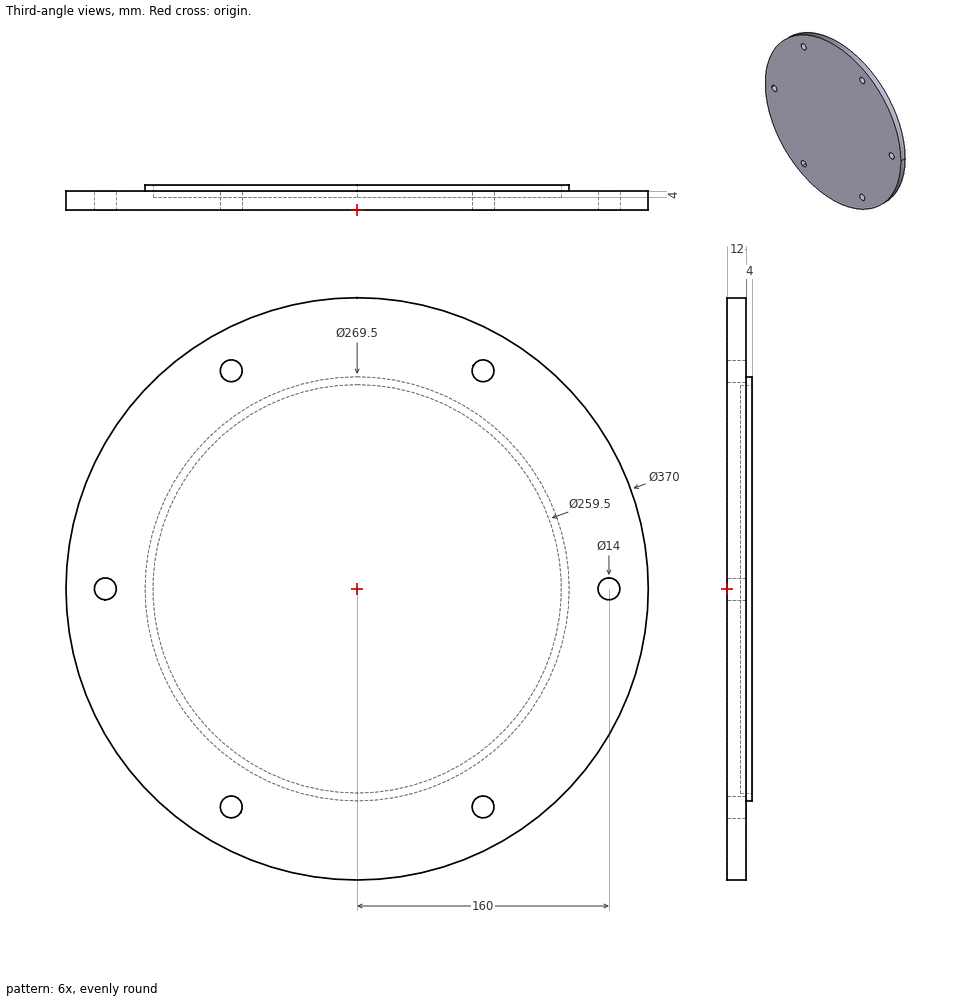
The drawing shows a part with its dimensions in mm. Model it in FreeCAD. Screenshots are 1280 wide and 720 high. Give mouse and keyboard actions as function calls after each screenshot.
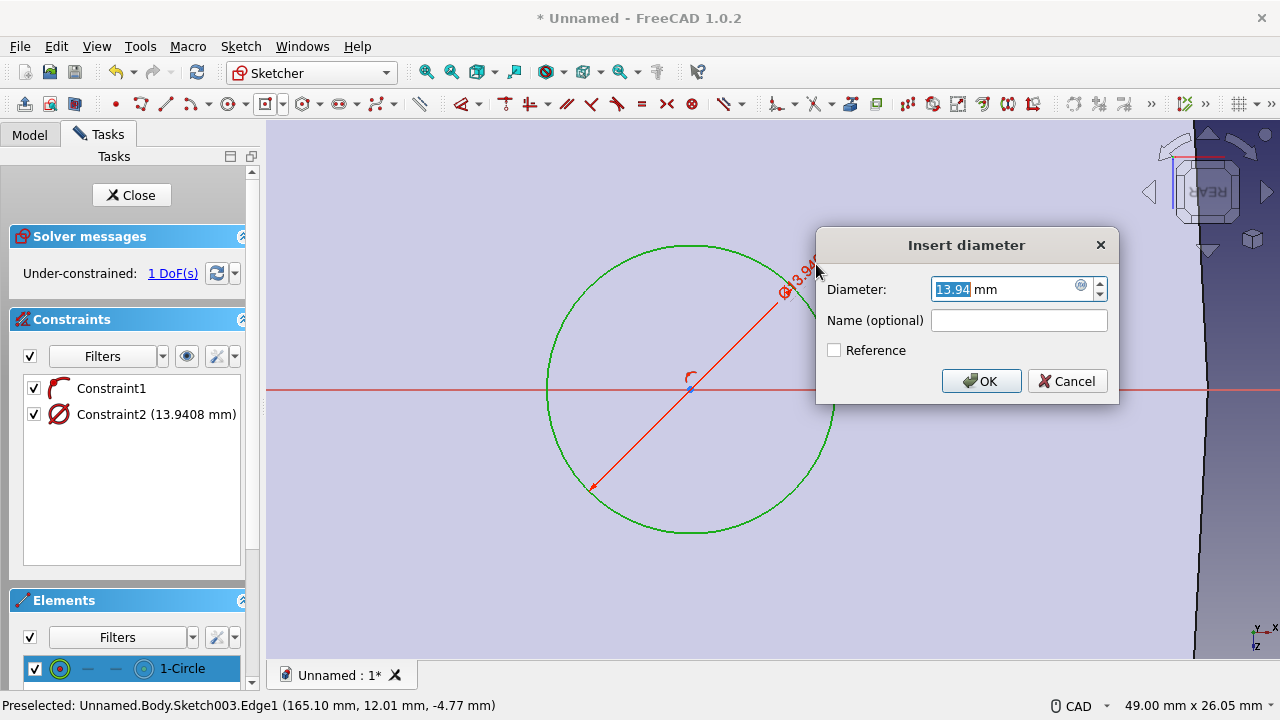
text(14)
key(Return)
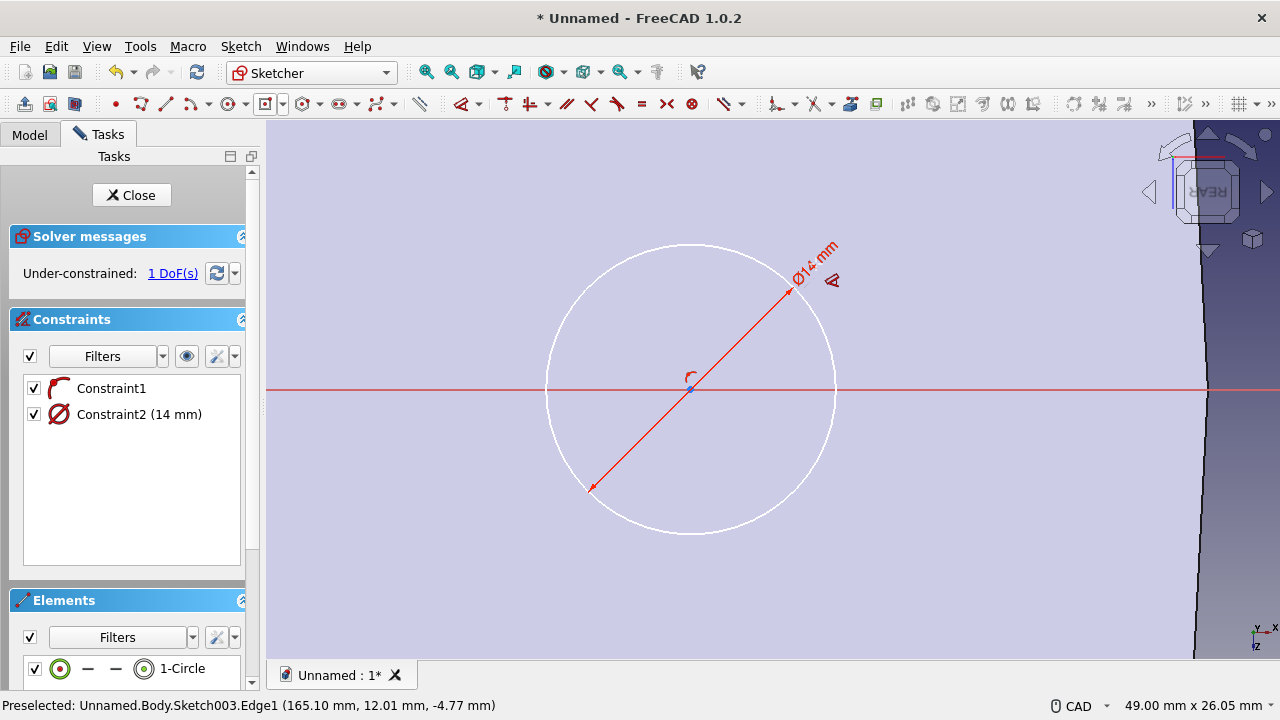
click(691, 389)
click(492, 423)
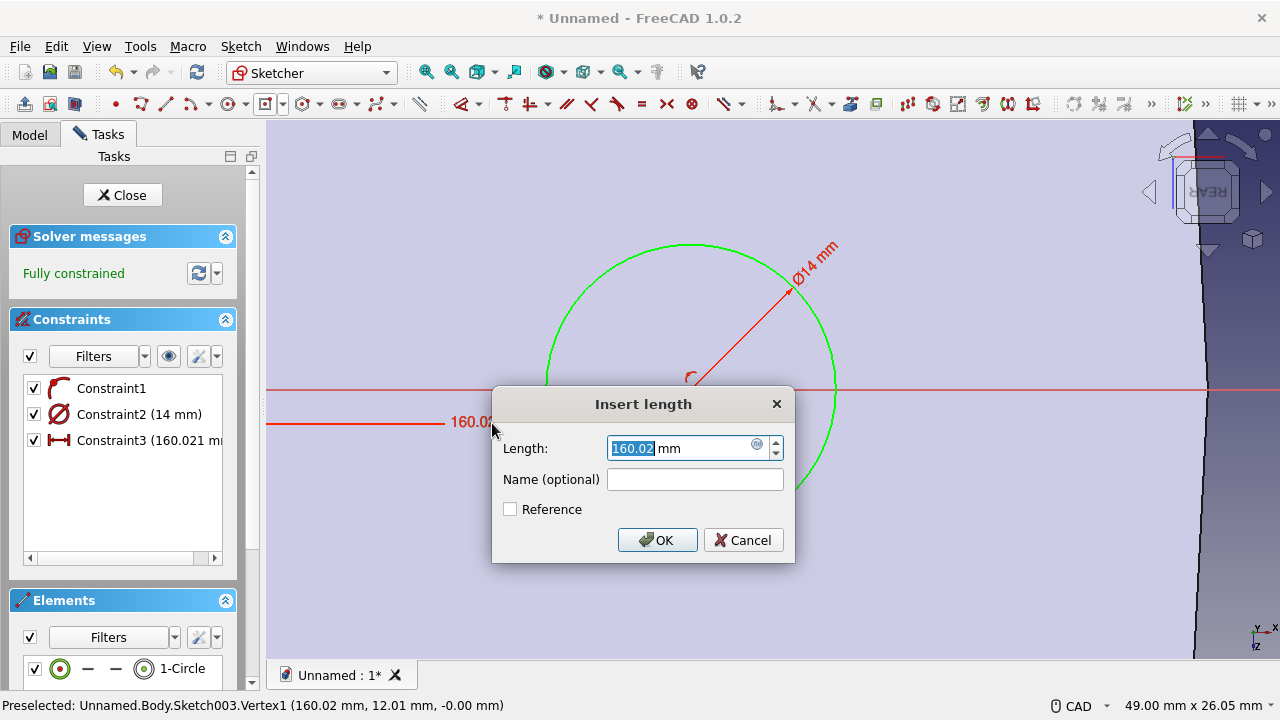
text(160)
key(Return)
key(Escape)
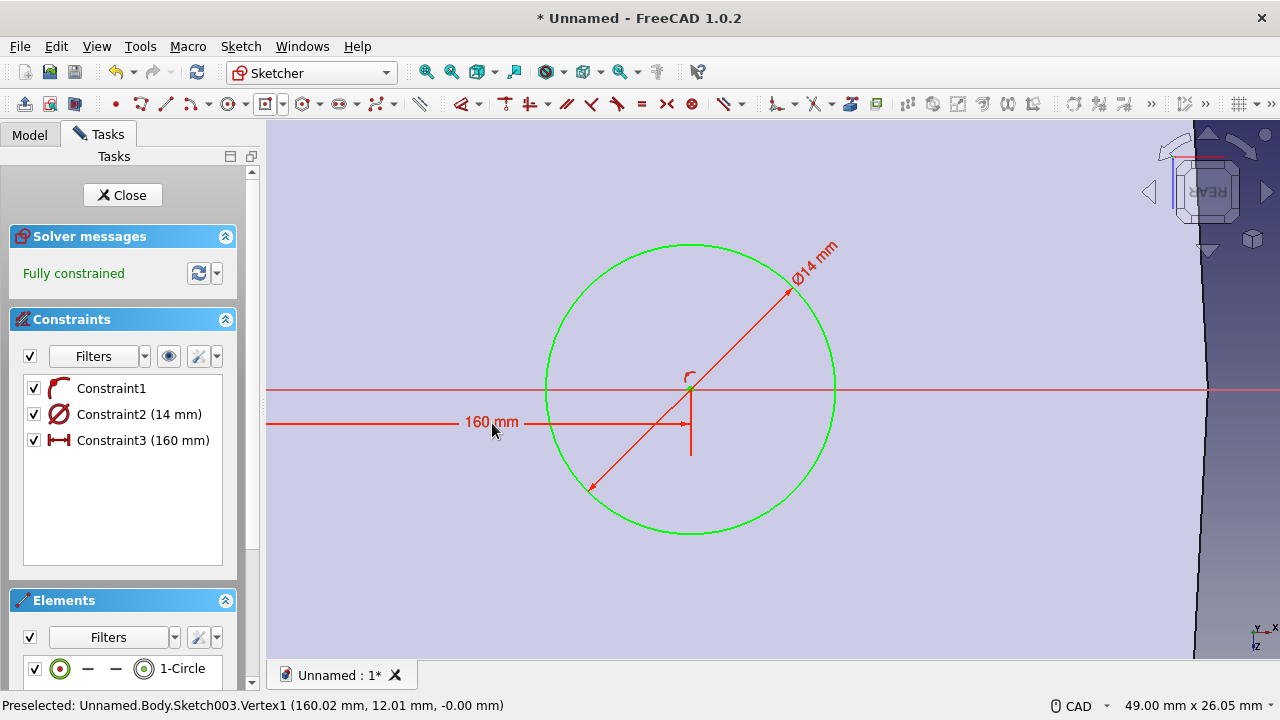
click(123, 195)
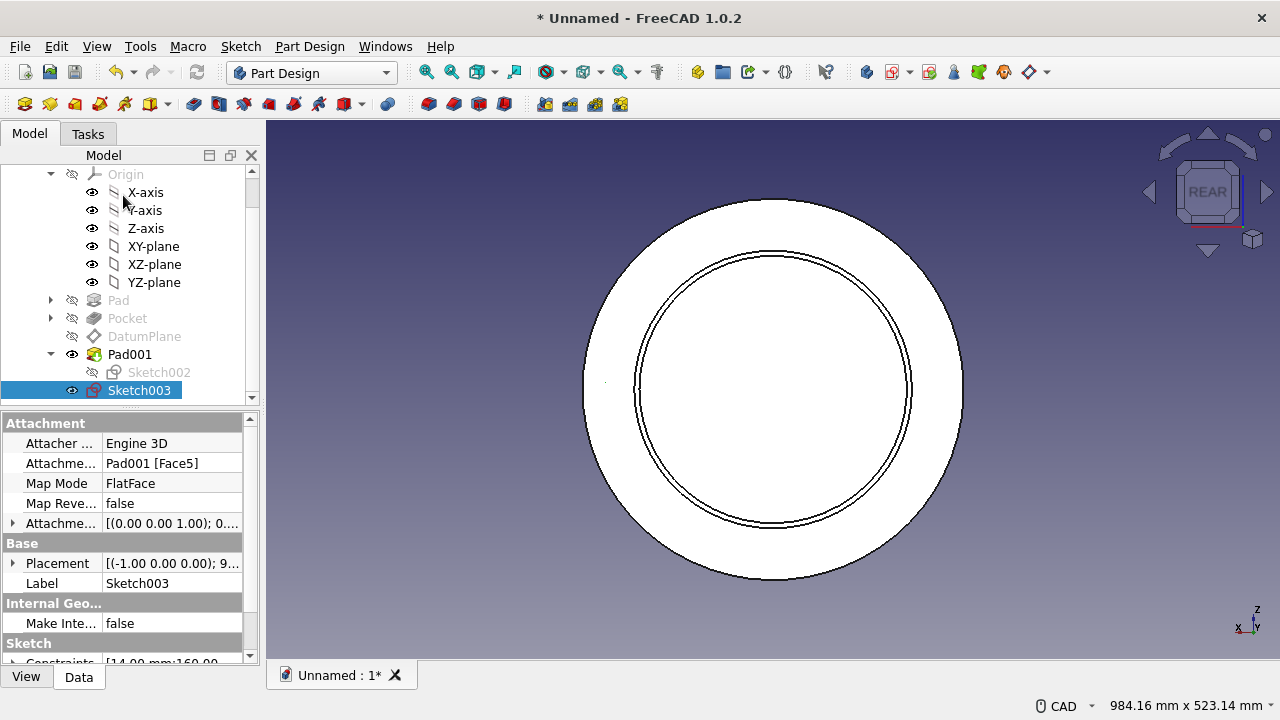
click(194, 104)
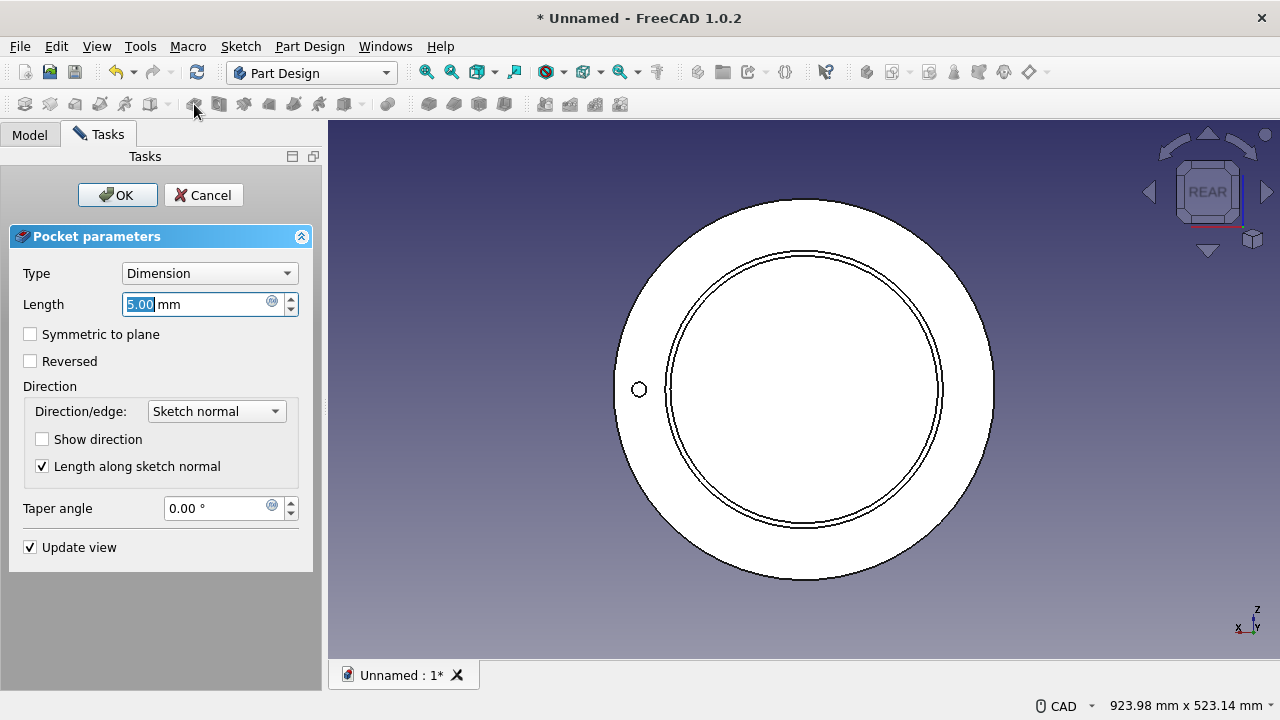
click(210, 274)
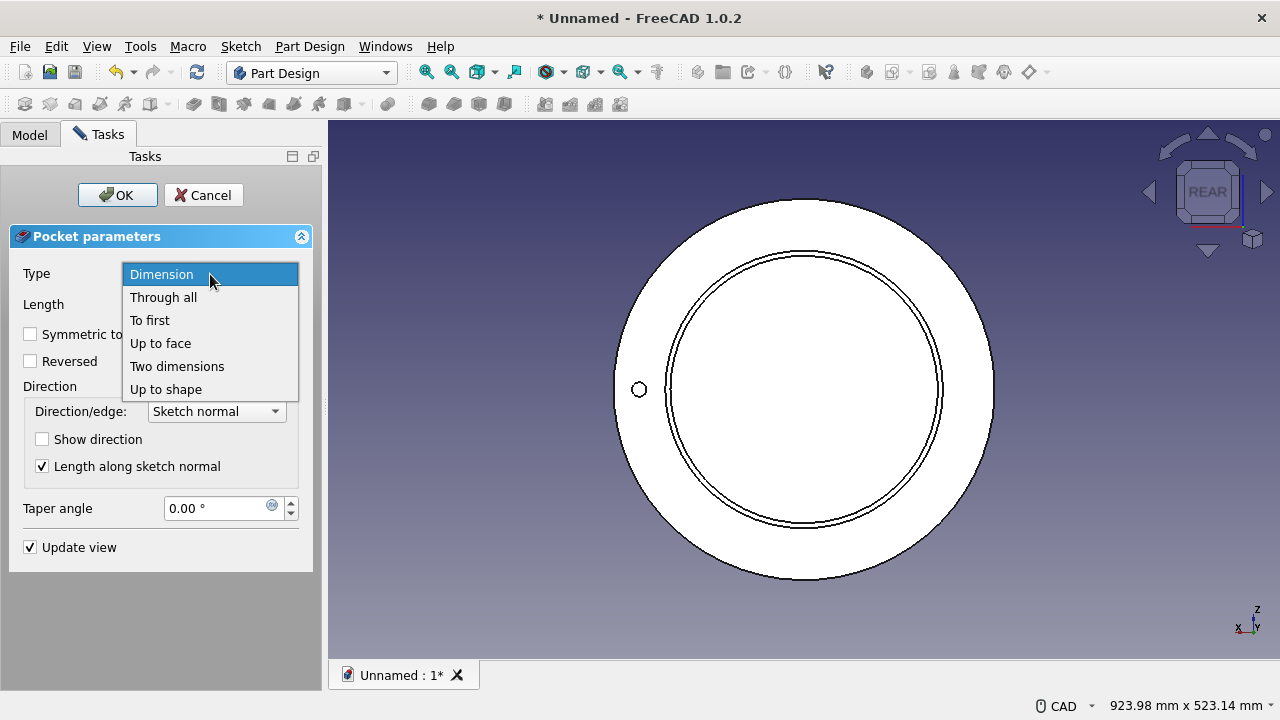
click(208, 298)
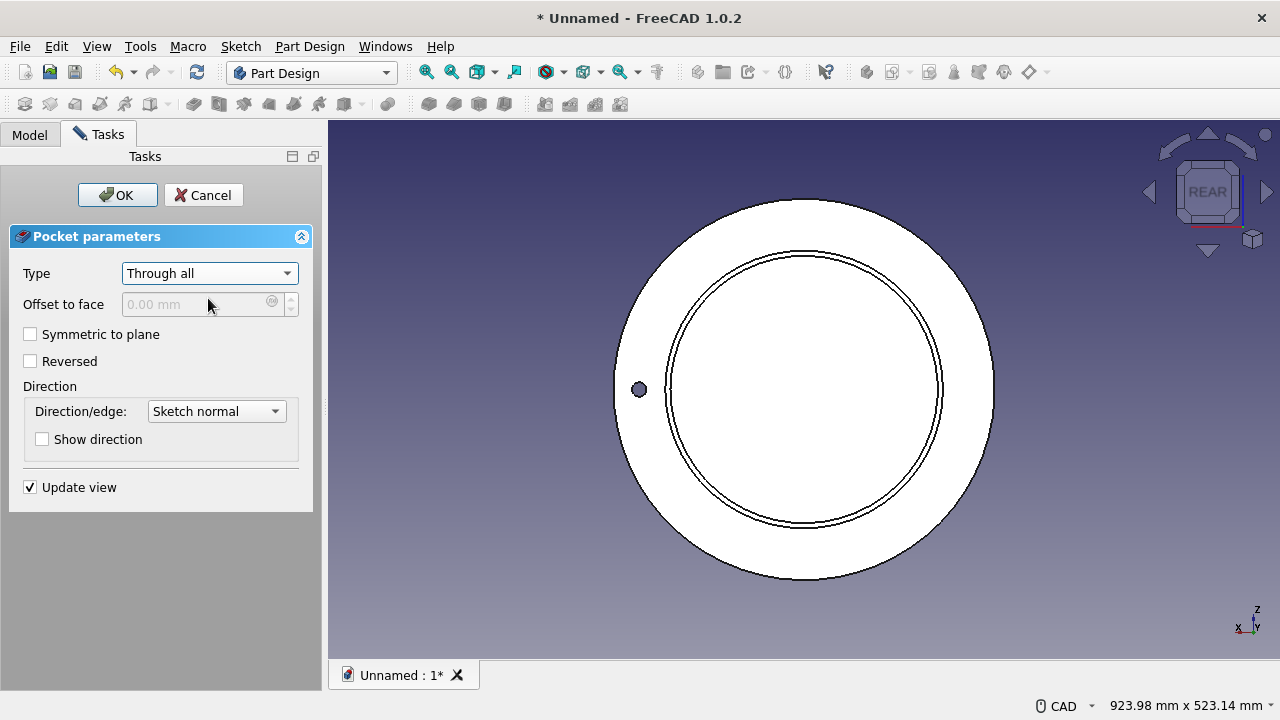
click(118, 195)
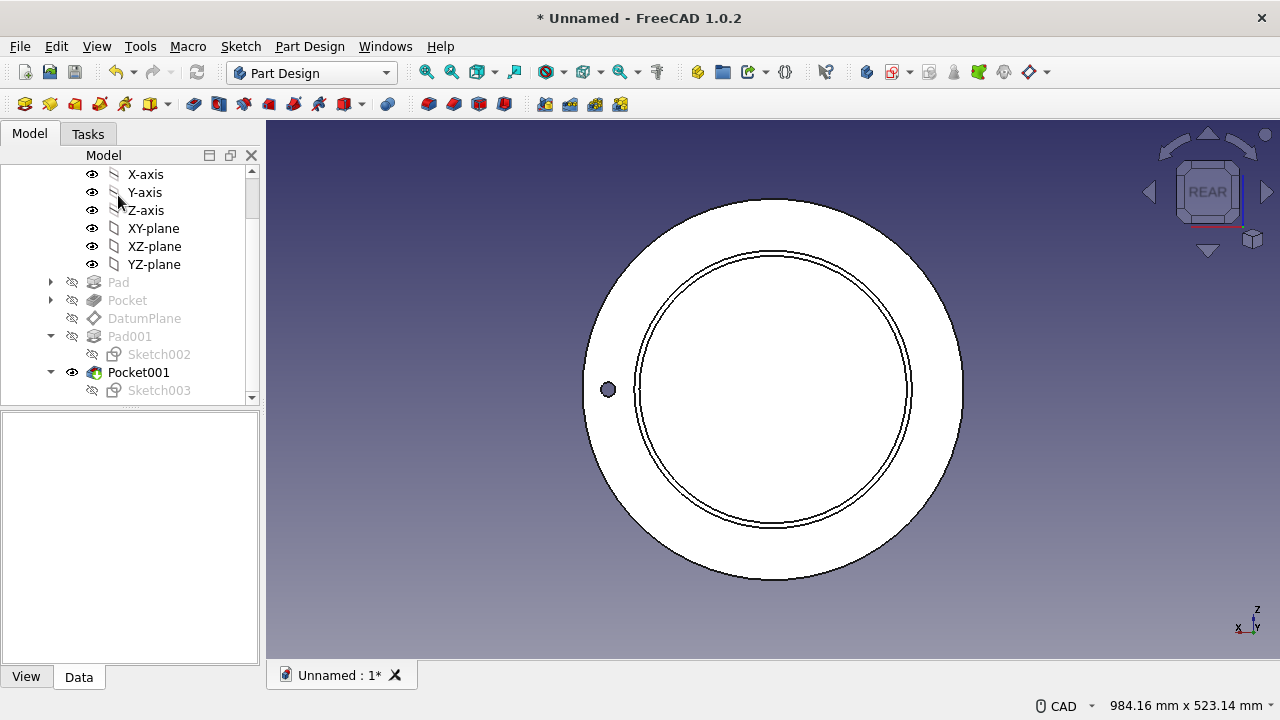
click(117, 372)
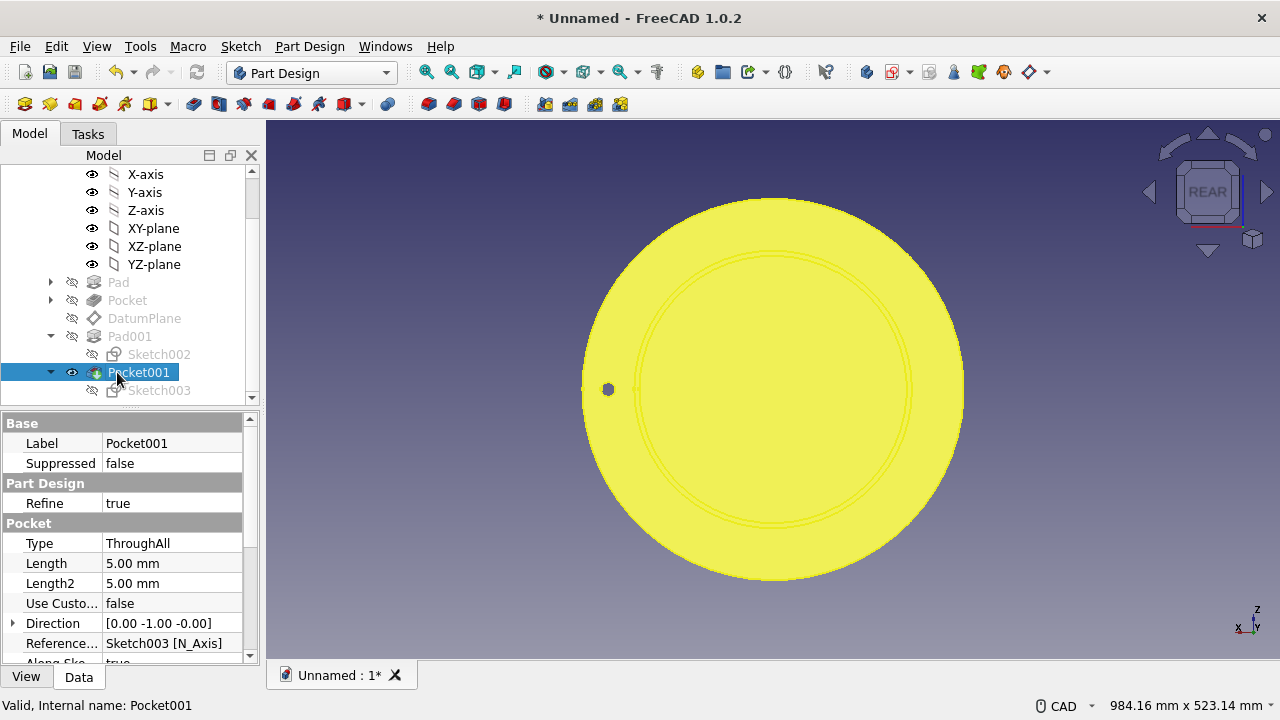
click(595, 104)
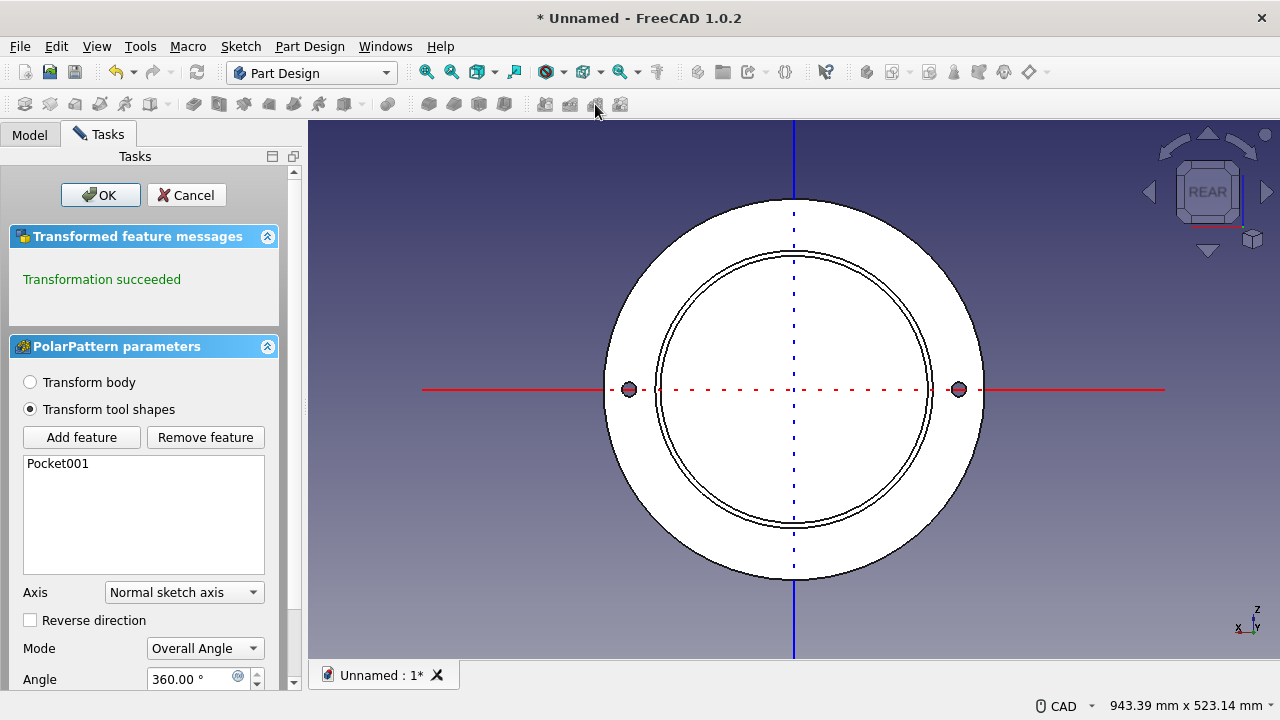
click(185, 592)